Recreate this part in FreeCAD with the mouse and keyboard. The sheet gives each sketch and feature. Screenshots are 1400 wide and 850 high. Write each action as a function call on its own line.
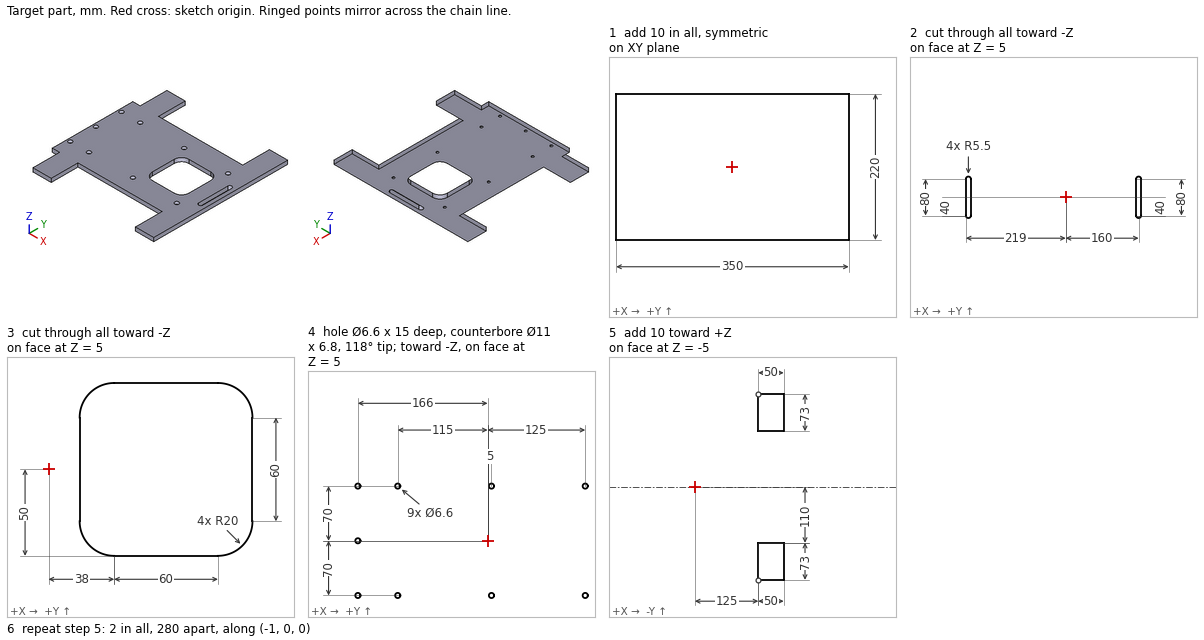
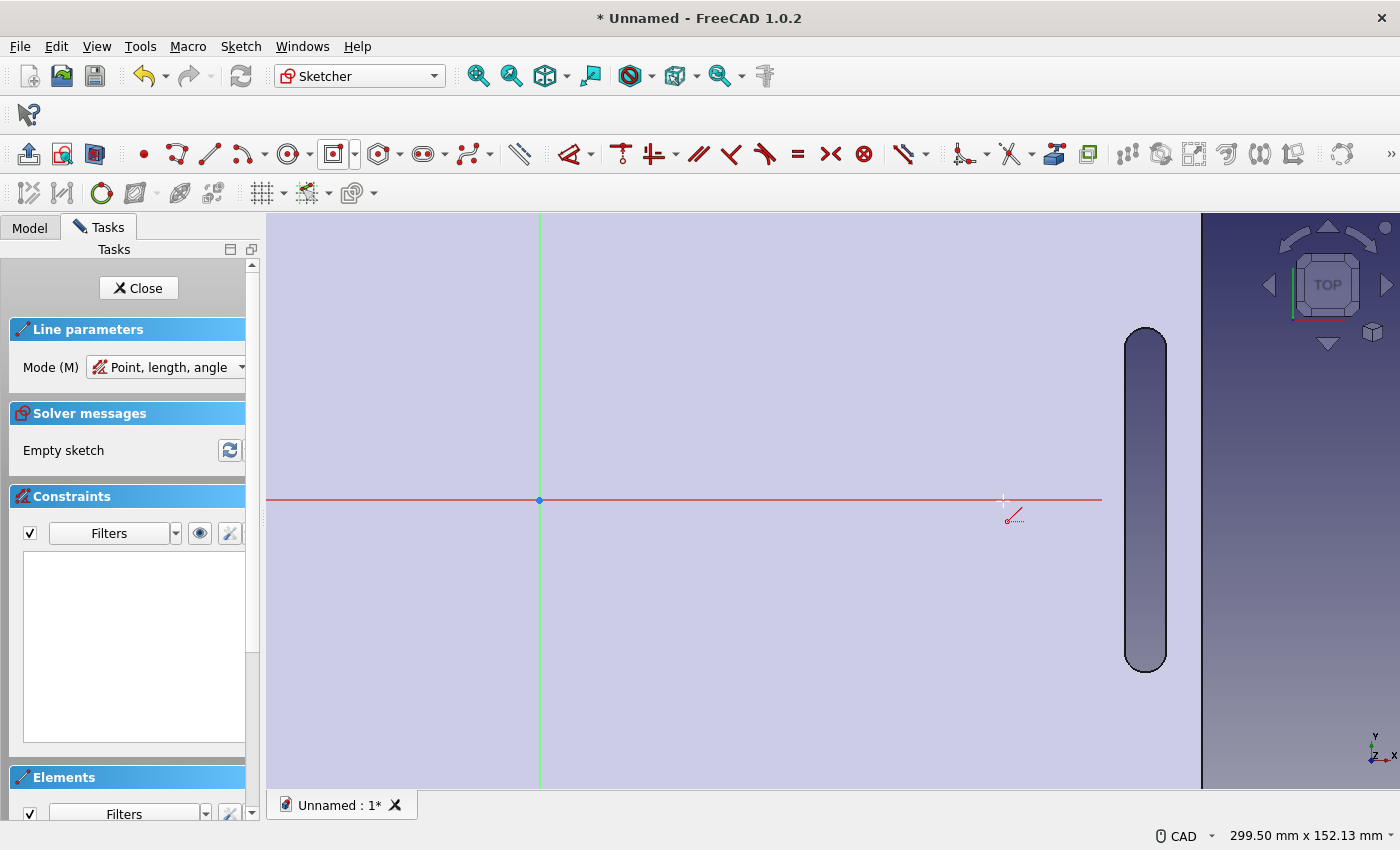
click(684, 689)
click(911, 689)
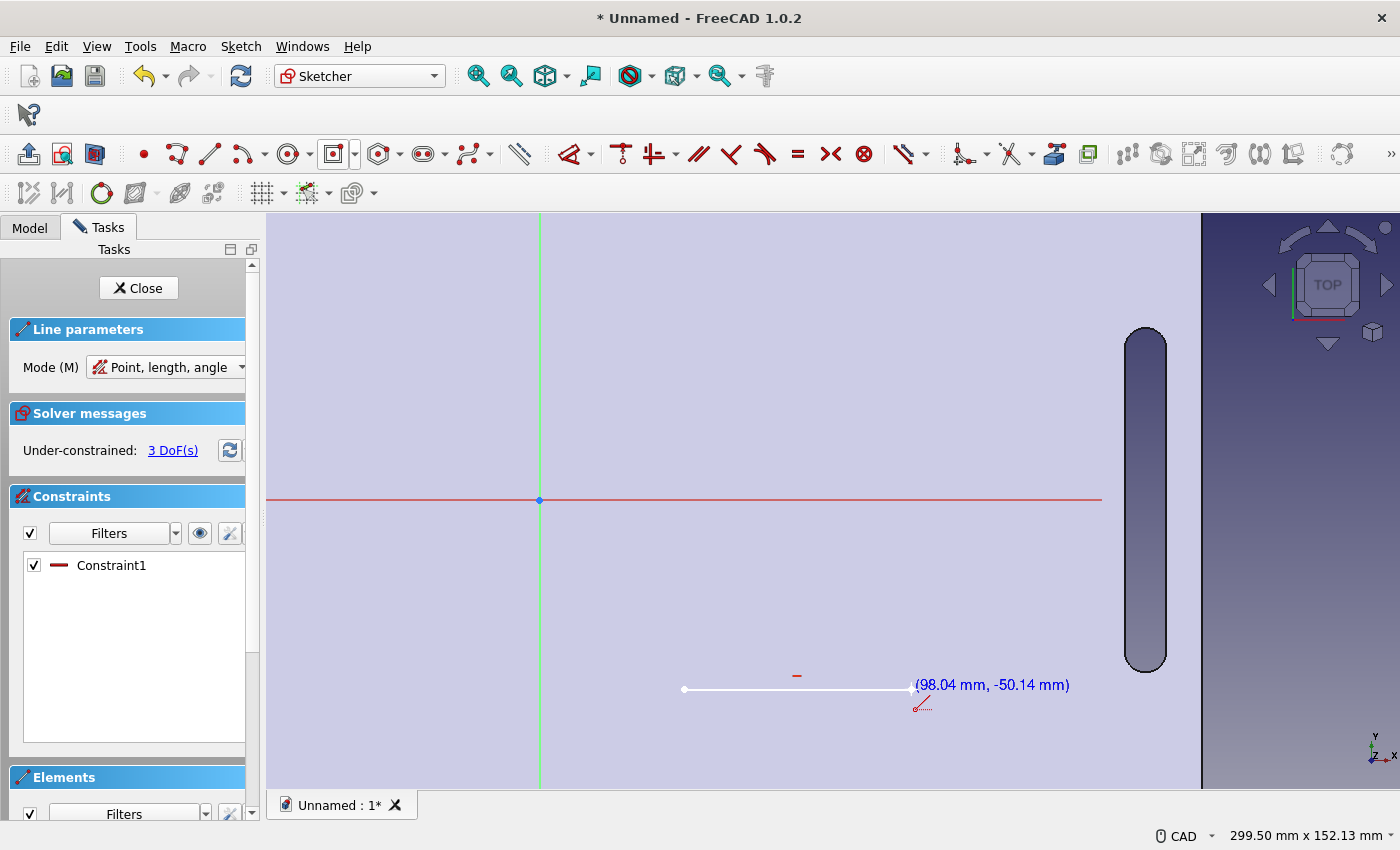
click(987, 614)
click(987, 387)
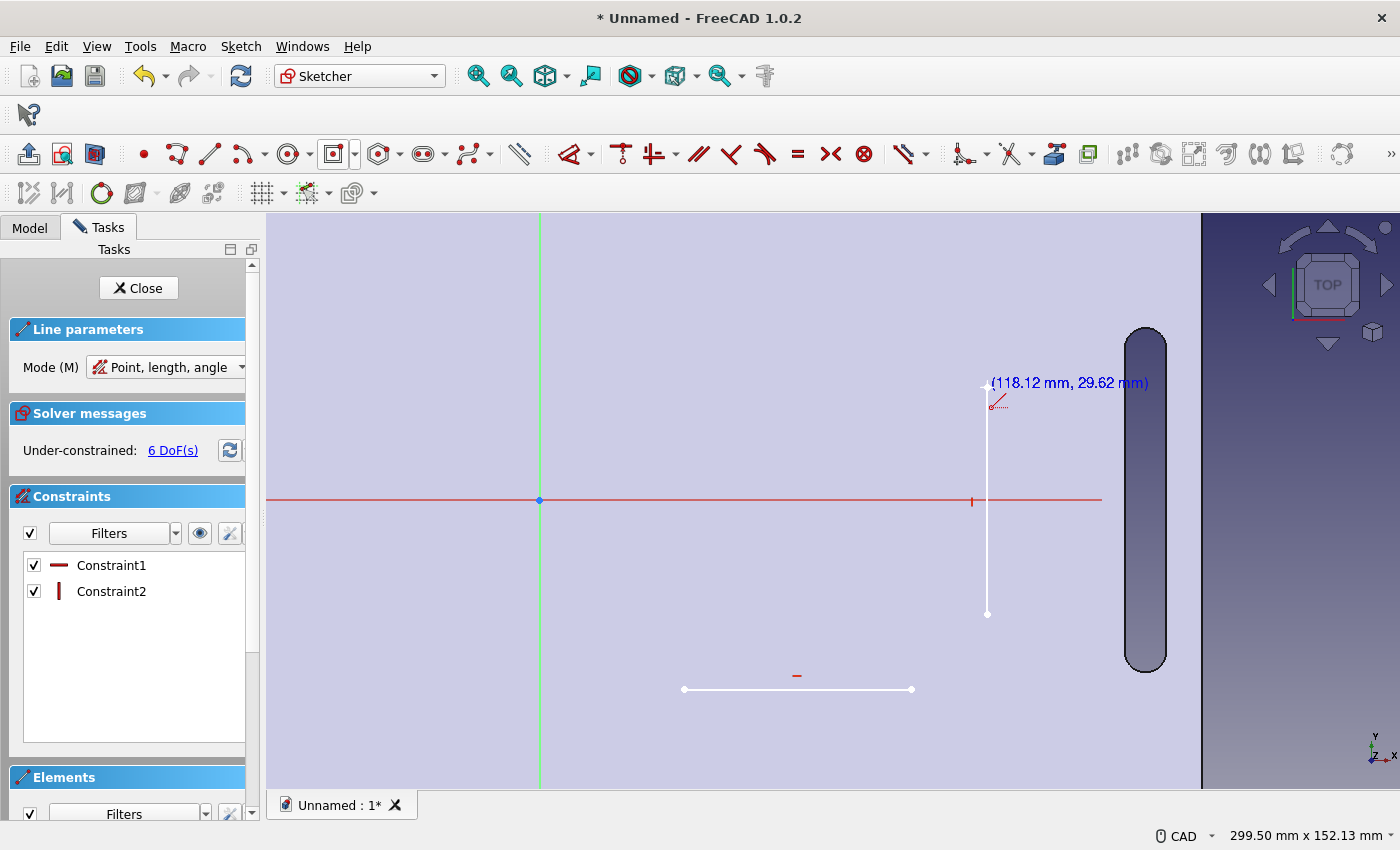
click(911, 311)
click(684, 311)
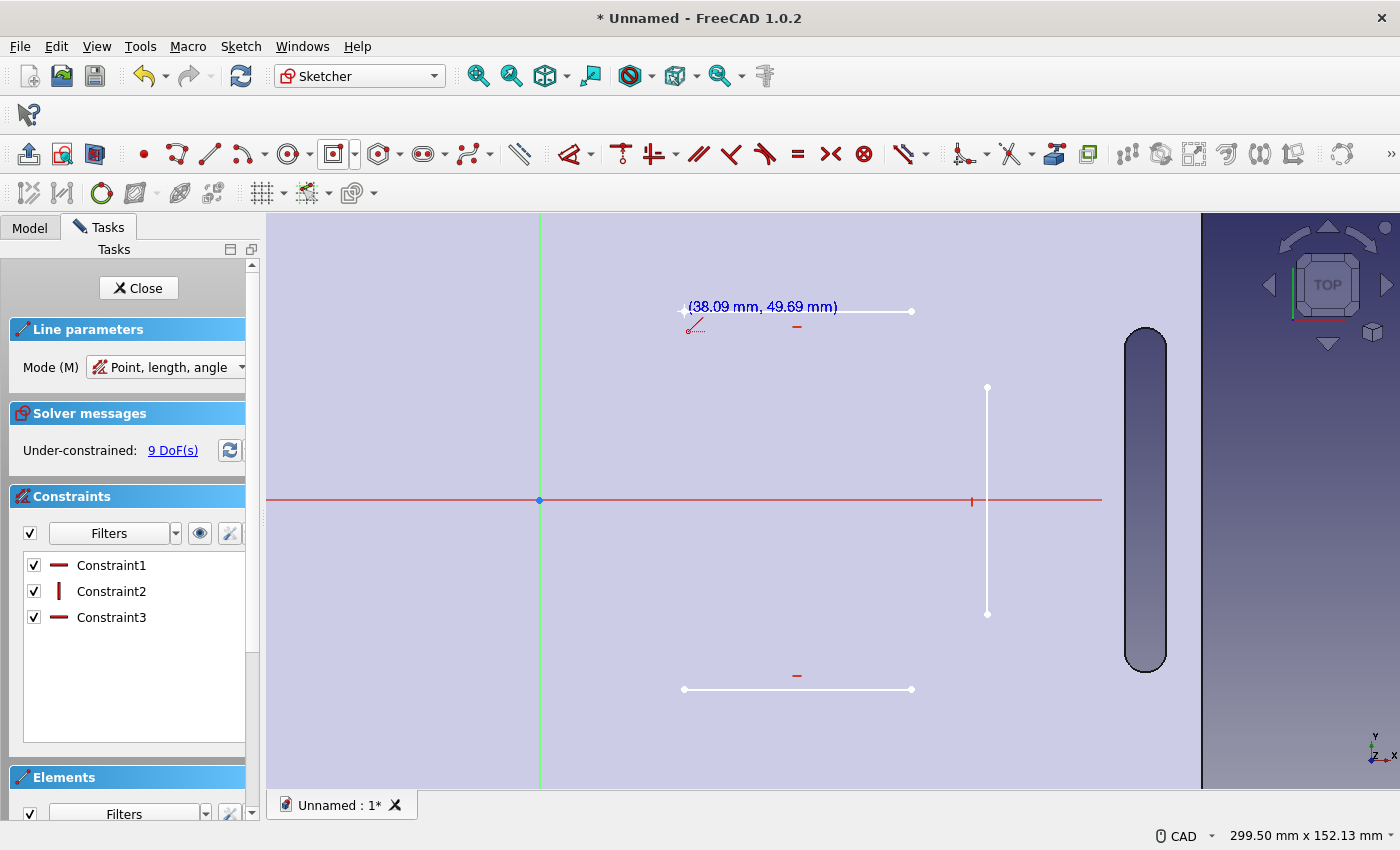
click(608, 387)
click(608, 614)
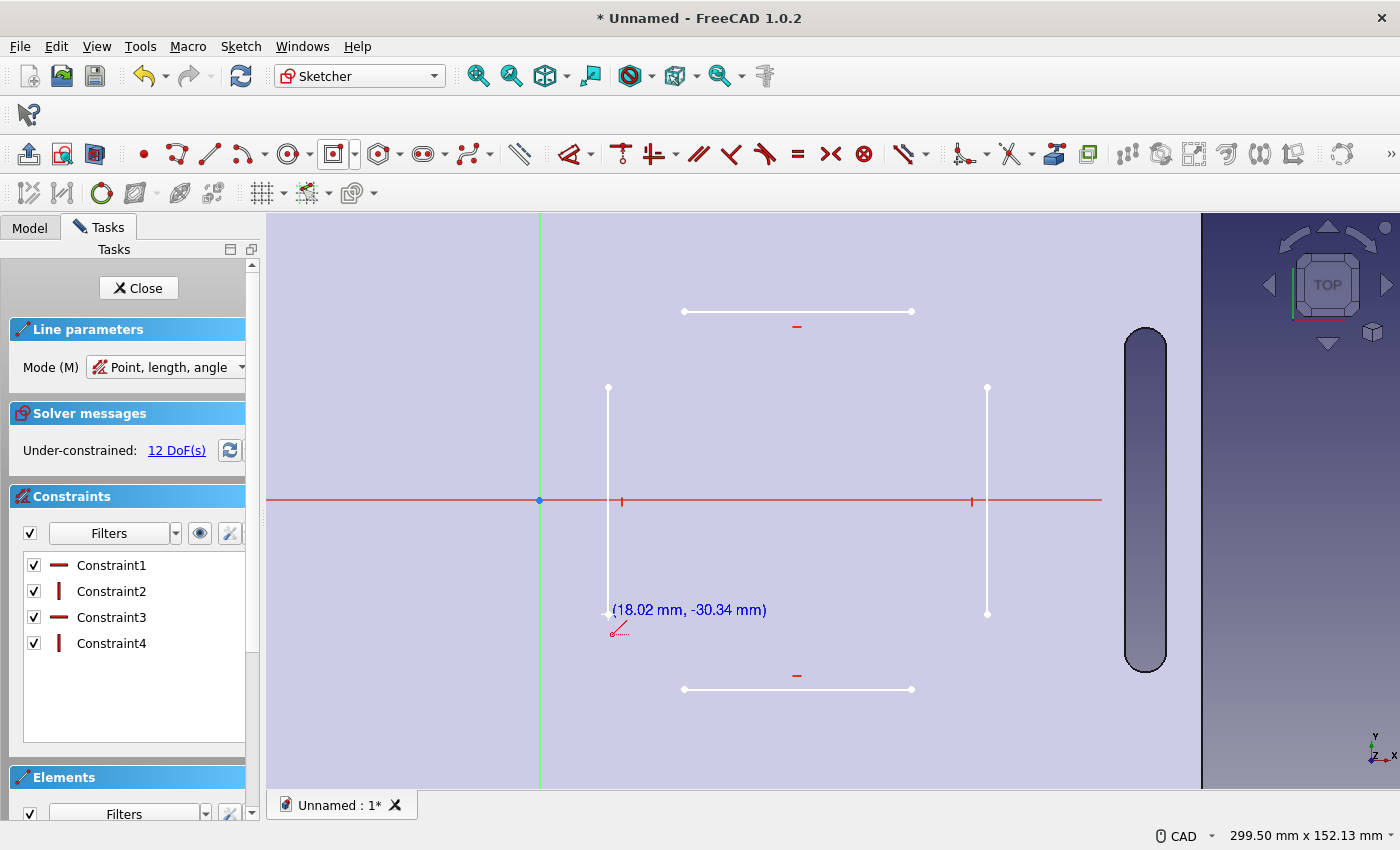
key(g)
key(3)
key(a)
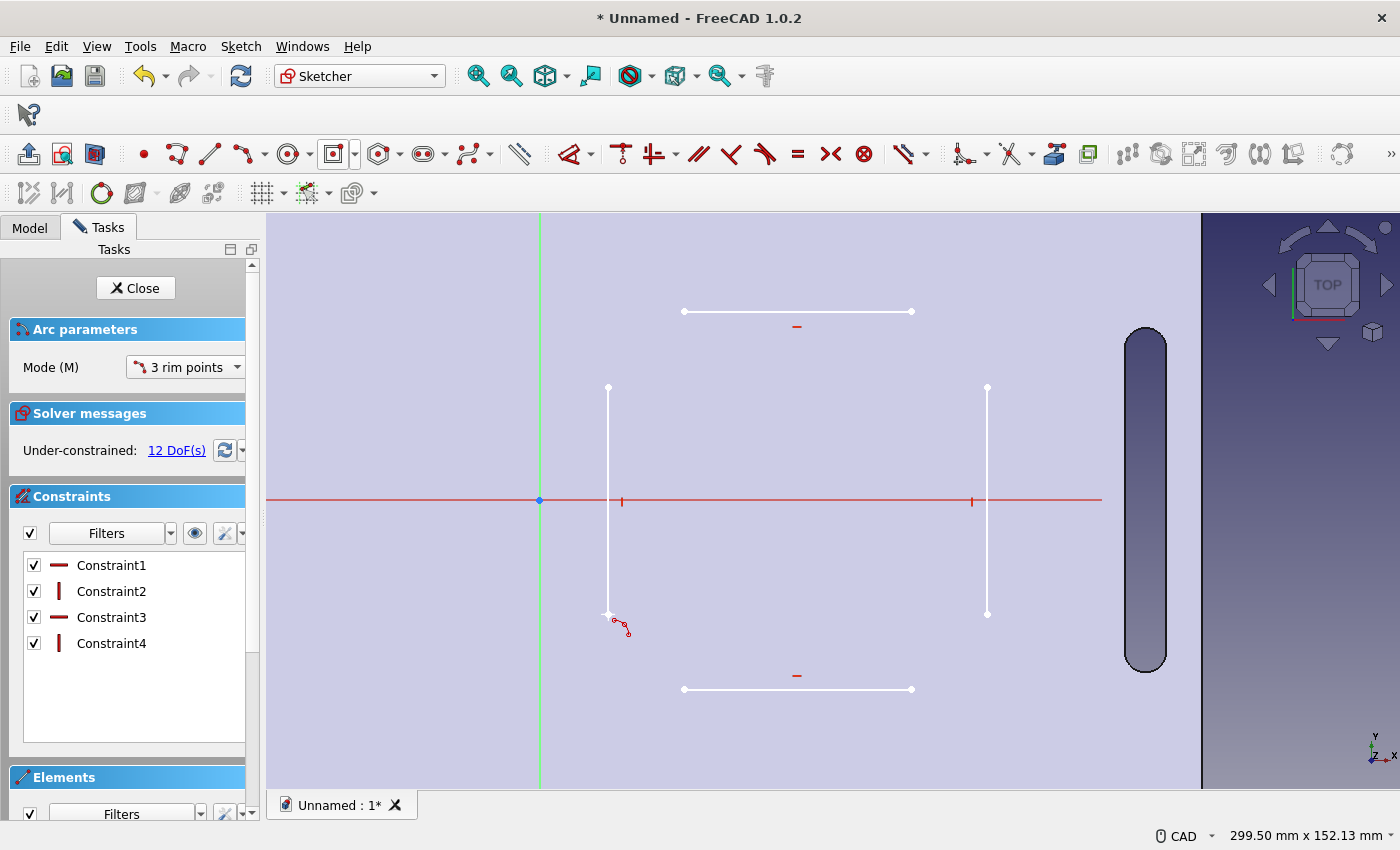
click(911, 690)
click(987, 615)
click(964, 667)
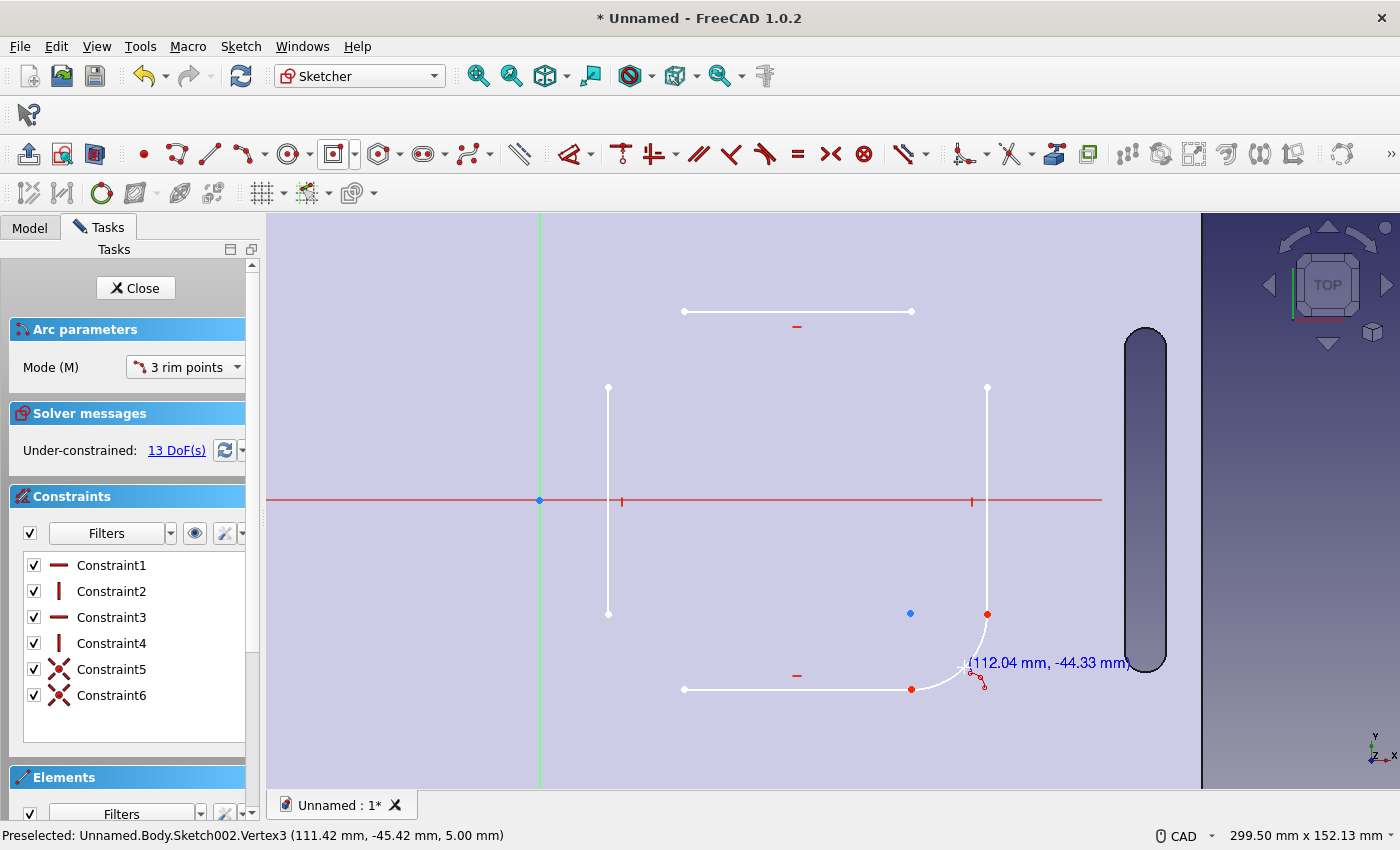
click(987, 388)
click(911, 312)
click(964, 333)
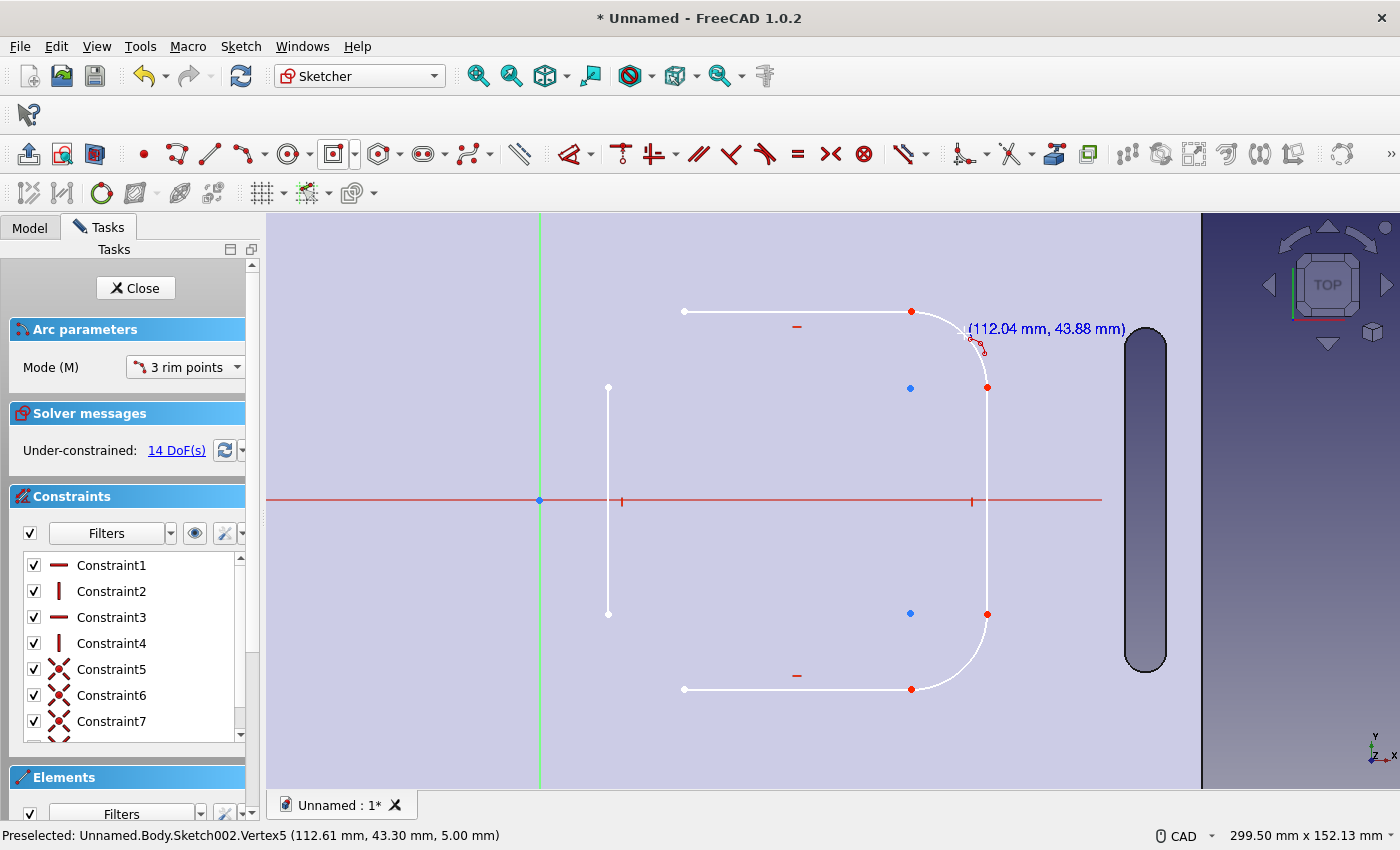
click(684, 312)
click(608, 388)
click(630, 333)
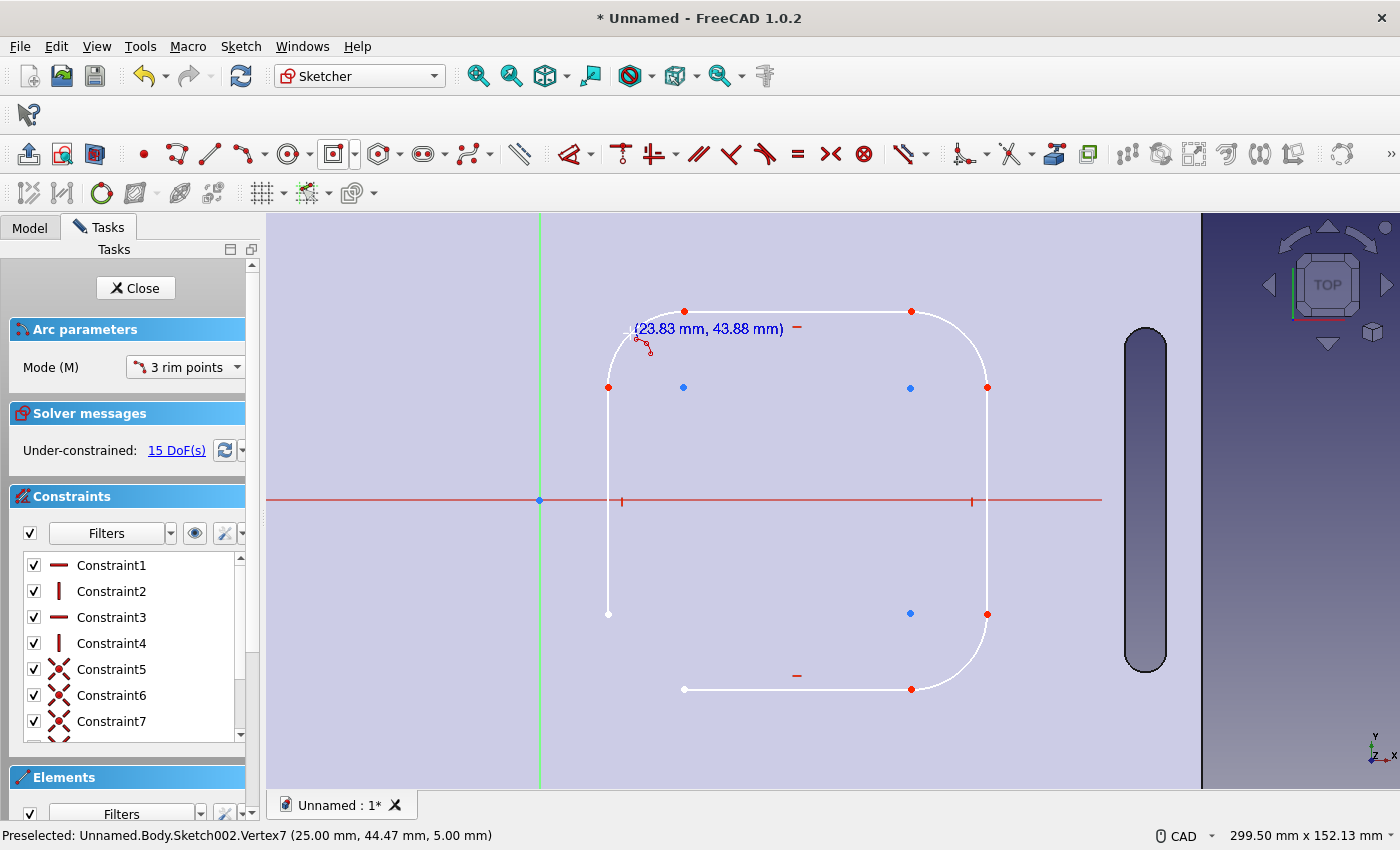
click(608, 615)
click(684, 690)
click(630, 667)
key(Escape)